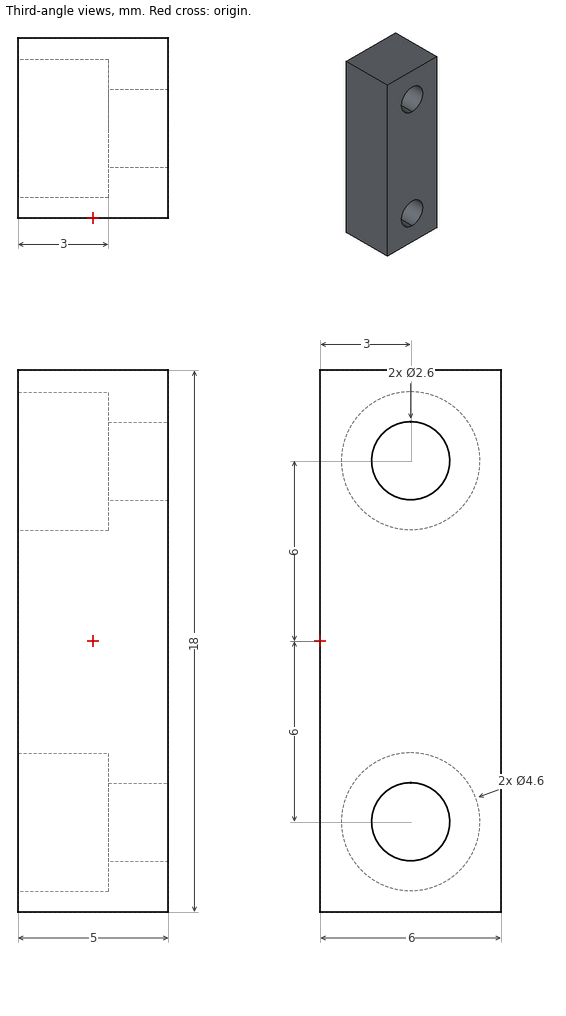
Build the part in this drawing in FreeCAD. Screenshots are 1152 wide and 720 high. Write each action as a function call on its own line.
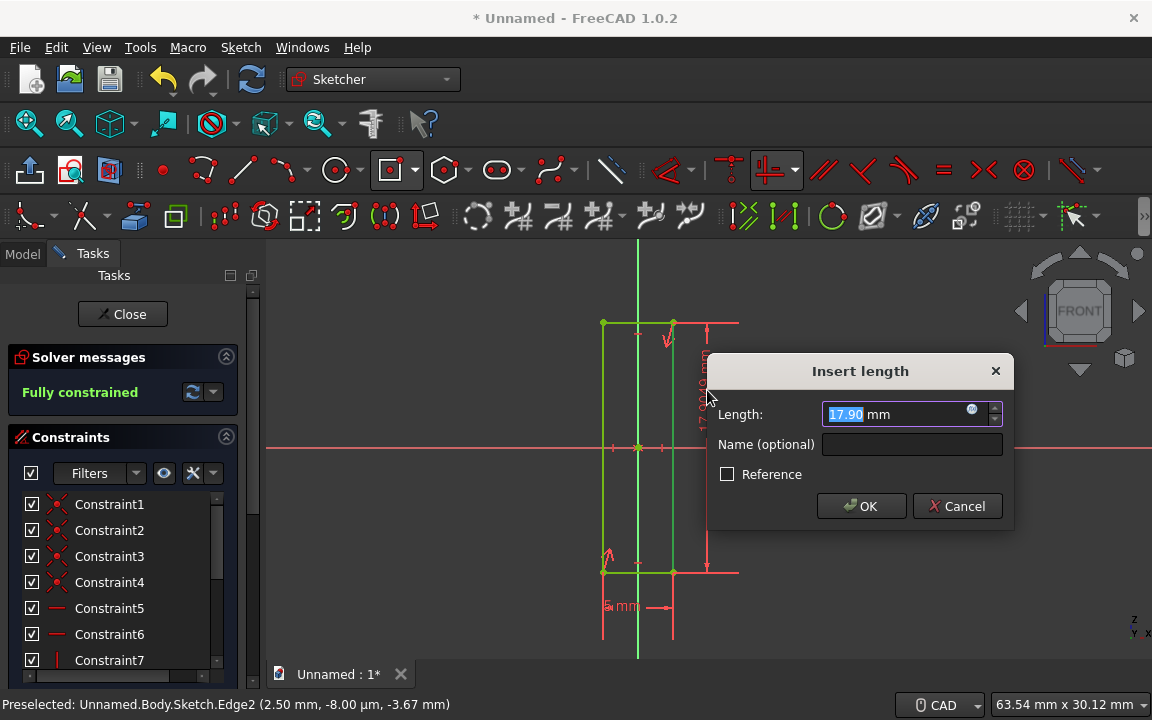
text(18)
key(Return)
key(Escape)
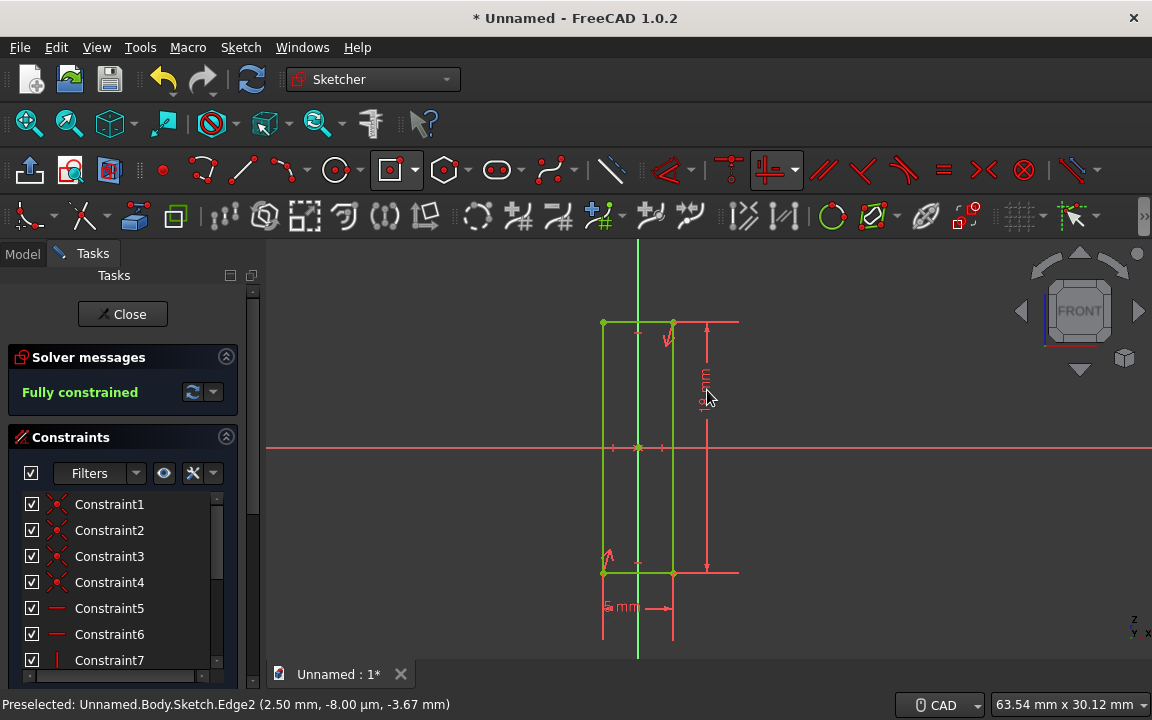
click(123, 314)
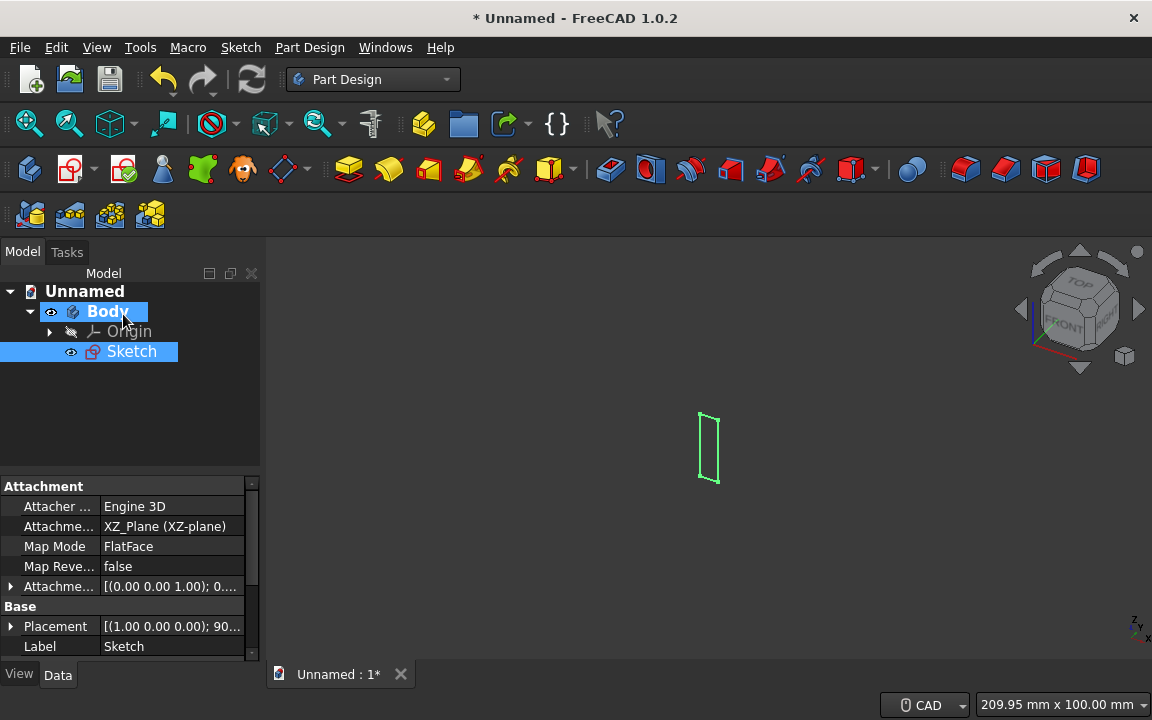
click(350, 170)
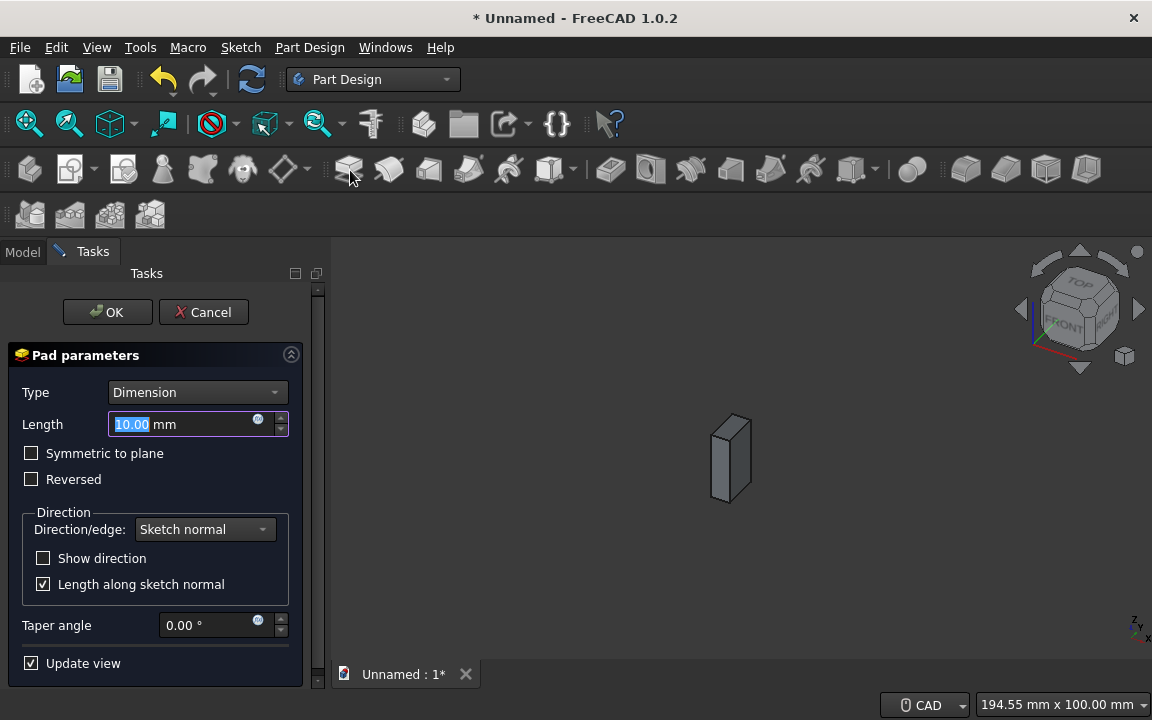
text(6)
key(Tab)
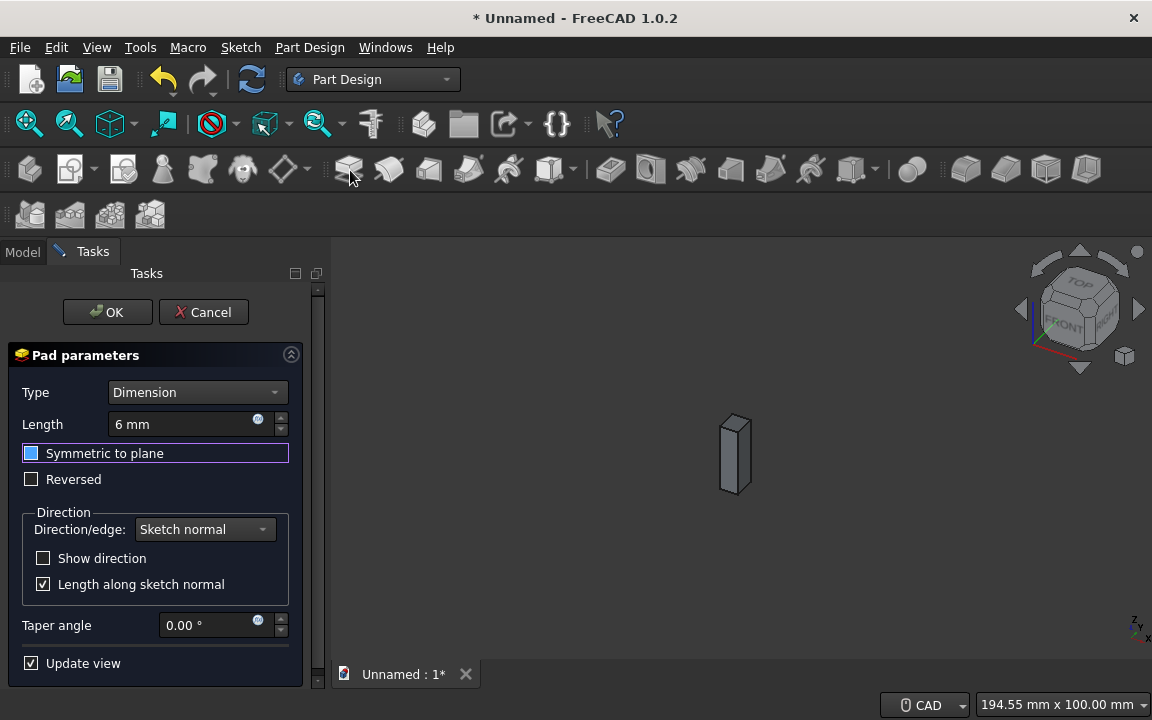
click(30, 479)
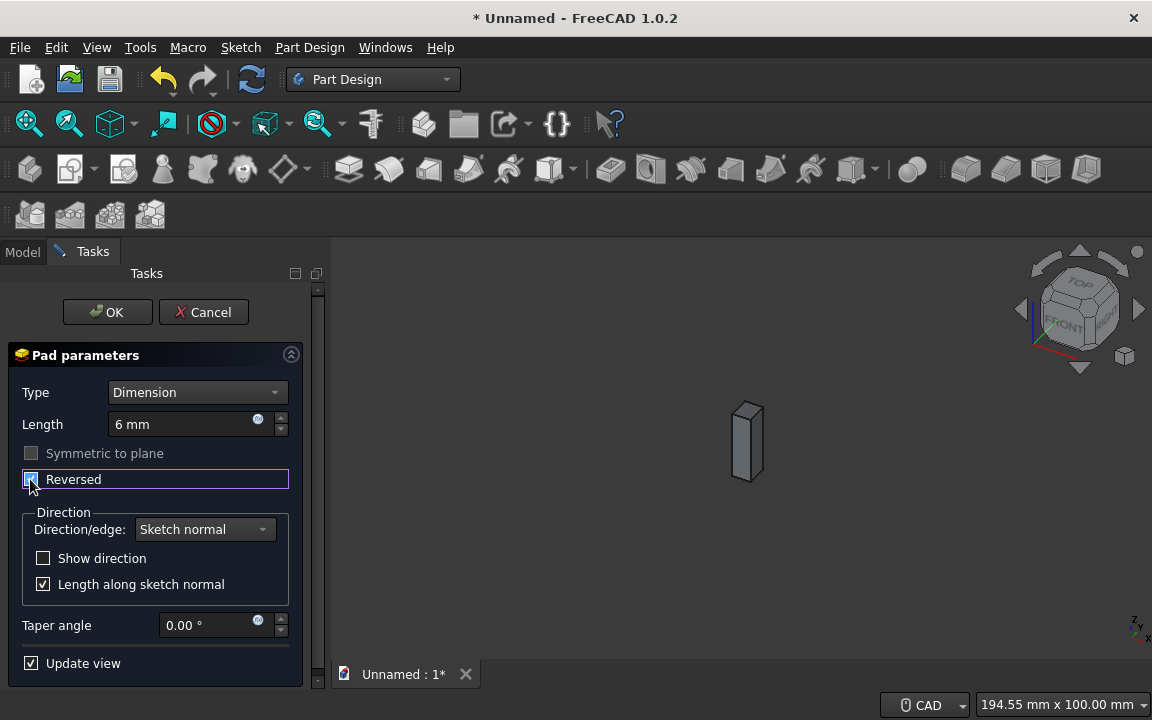
click(108, 312)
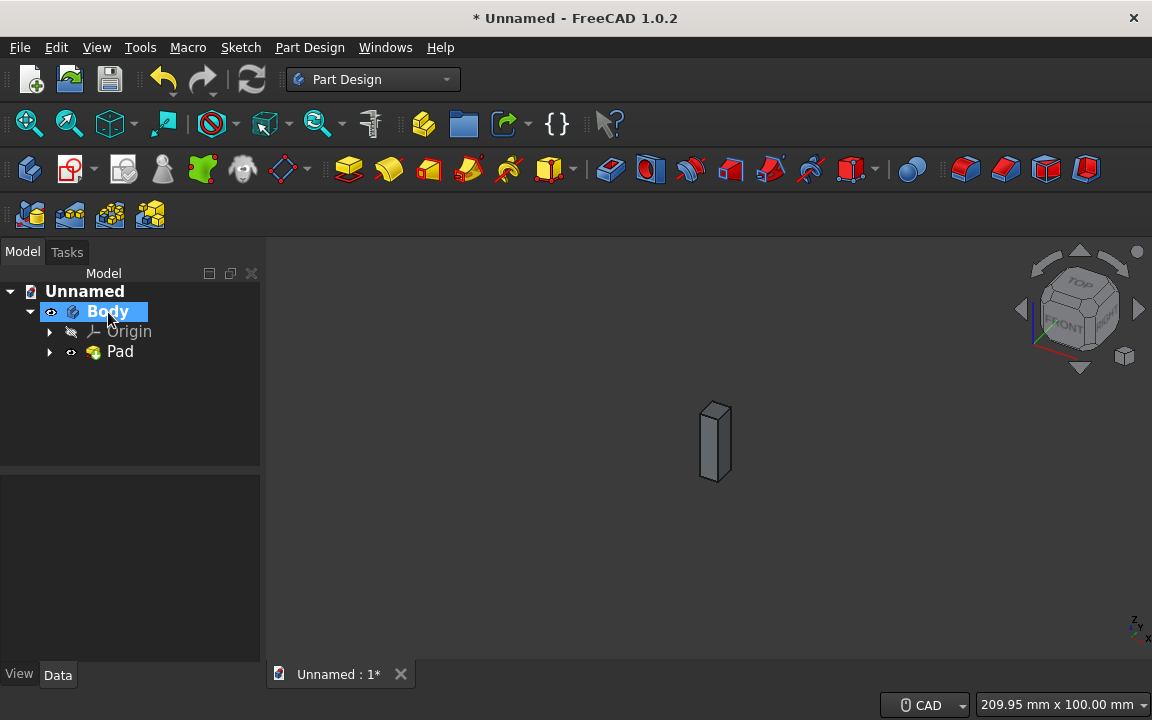
click(30, 124)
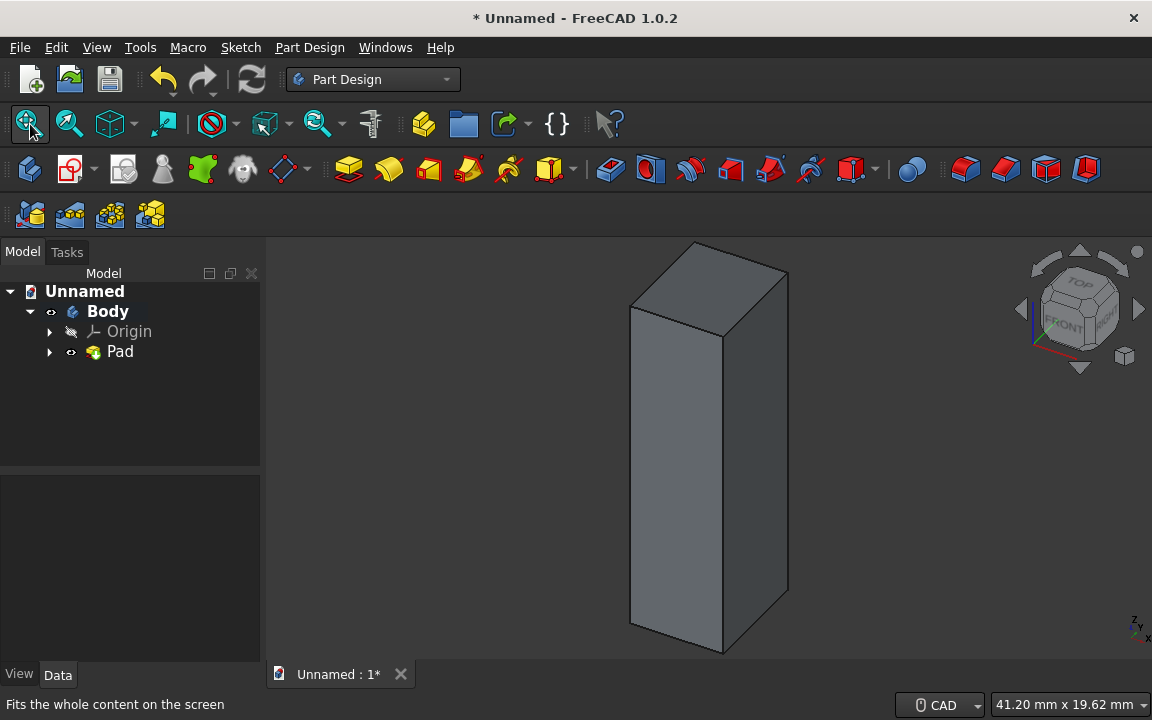
key(6)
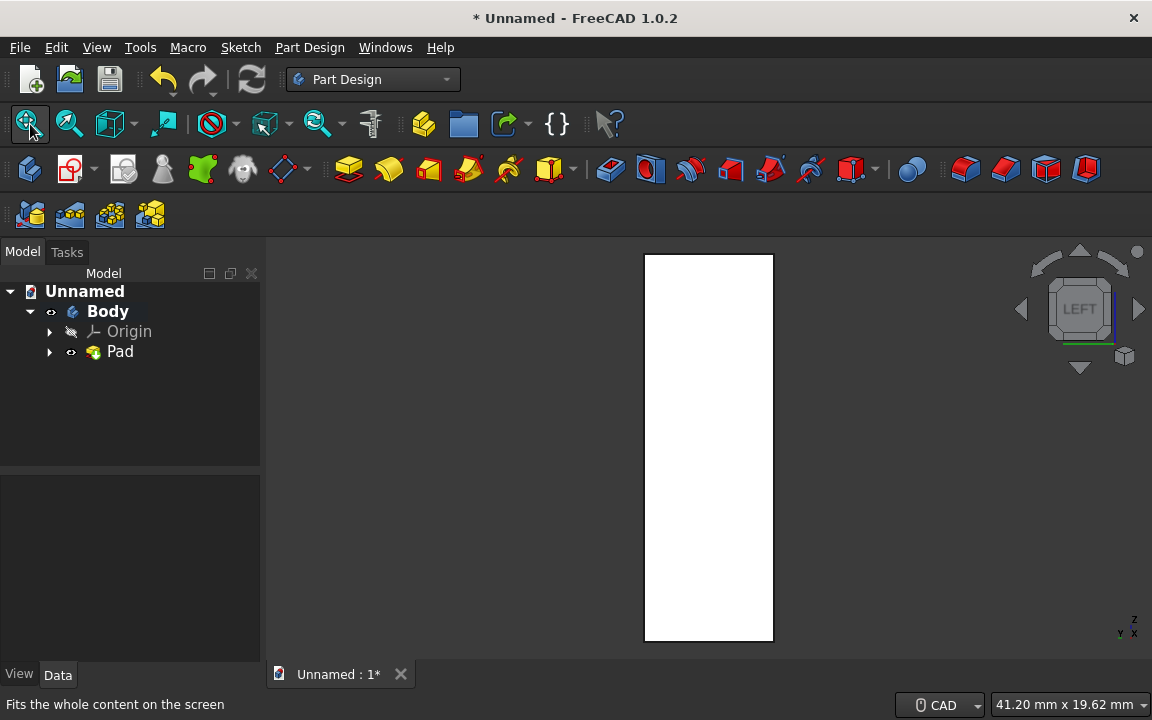
click(709, 447)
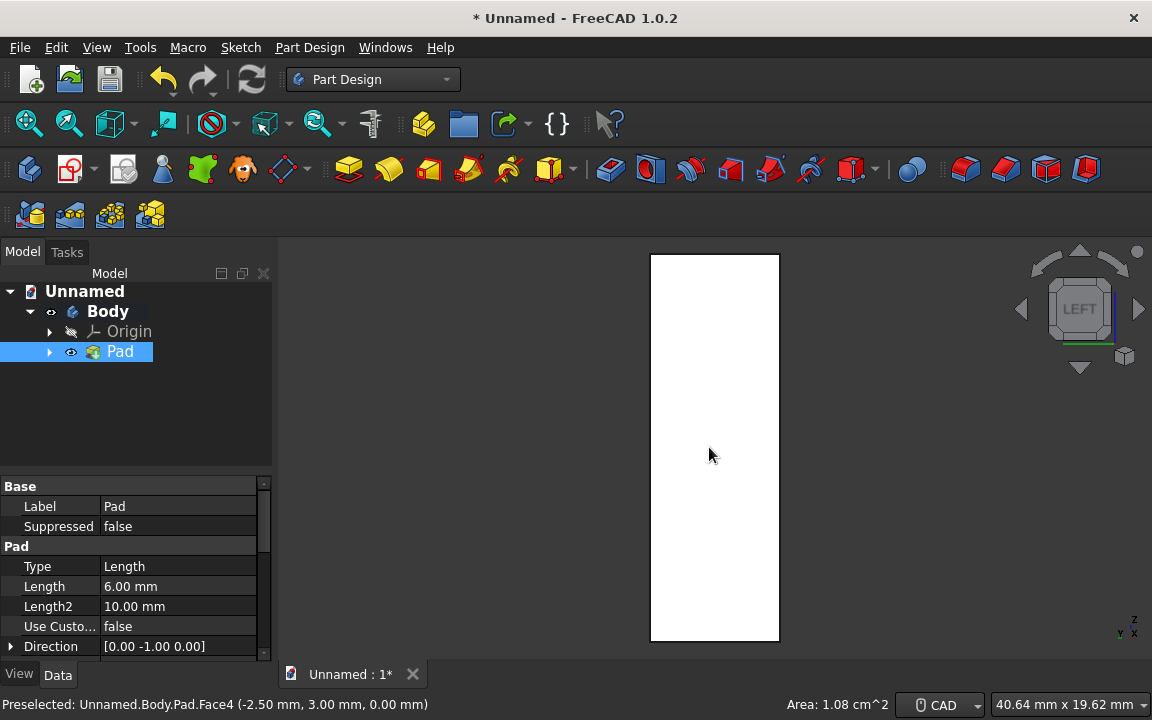
click(70, 170)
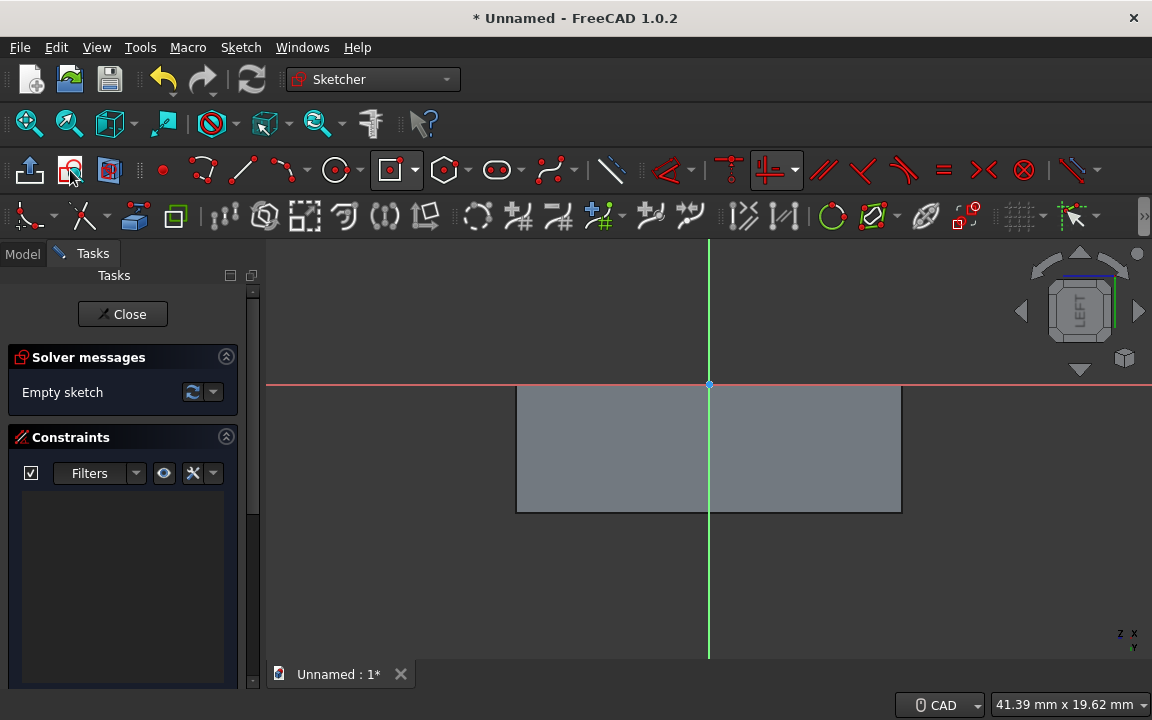
scroll(848, 394, up, 2)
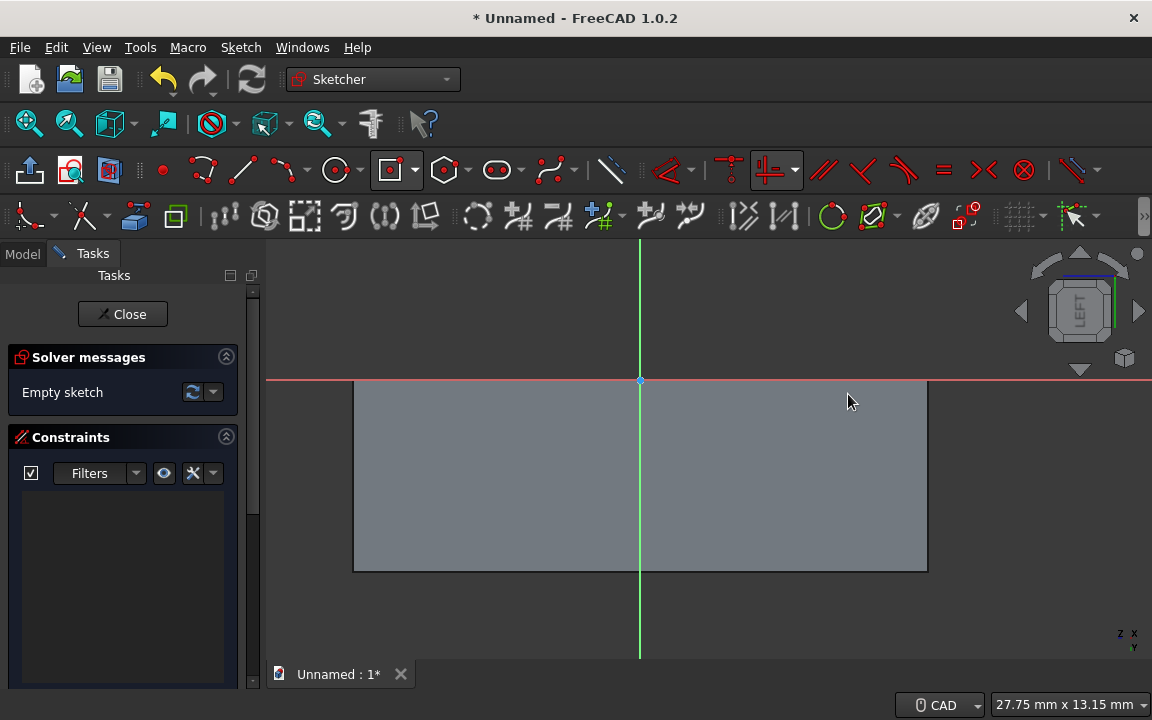
click(336, 170)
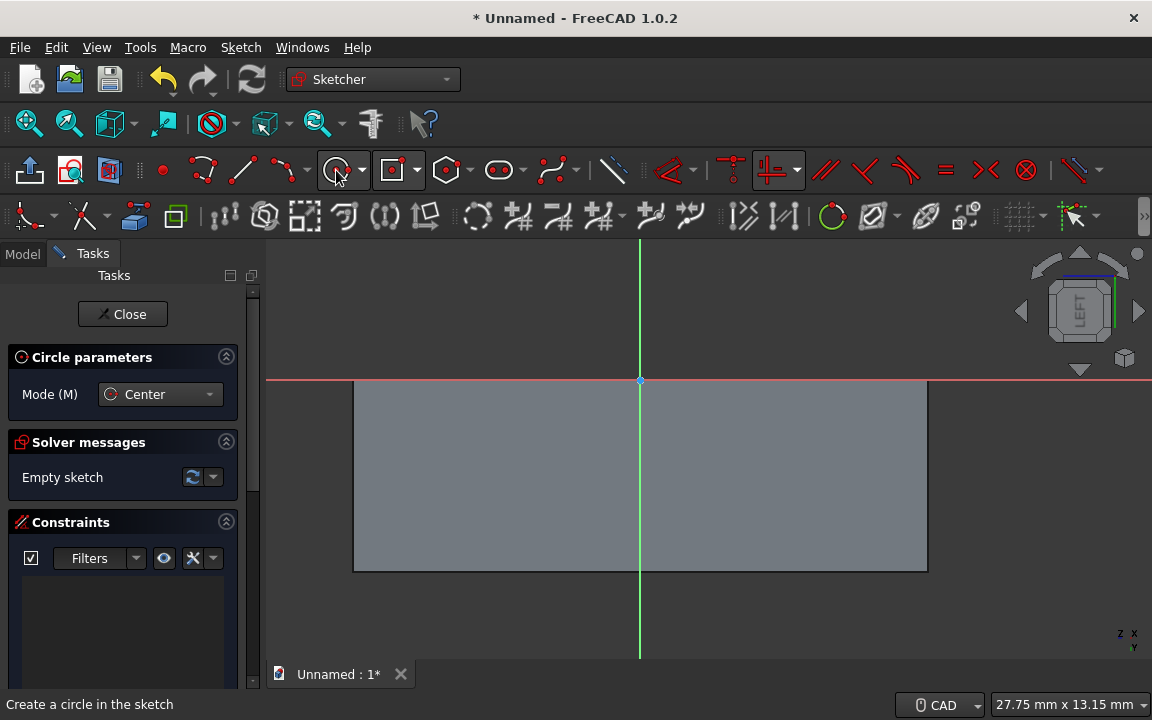
click(449, 476)
click(478, 447)